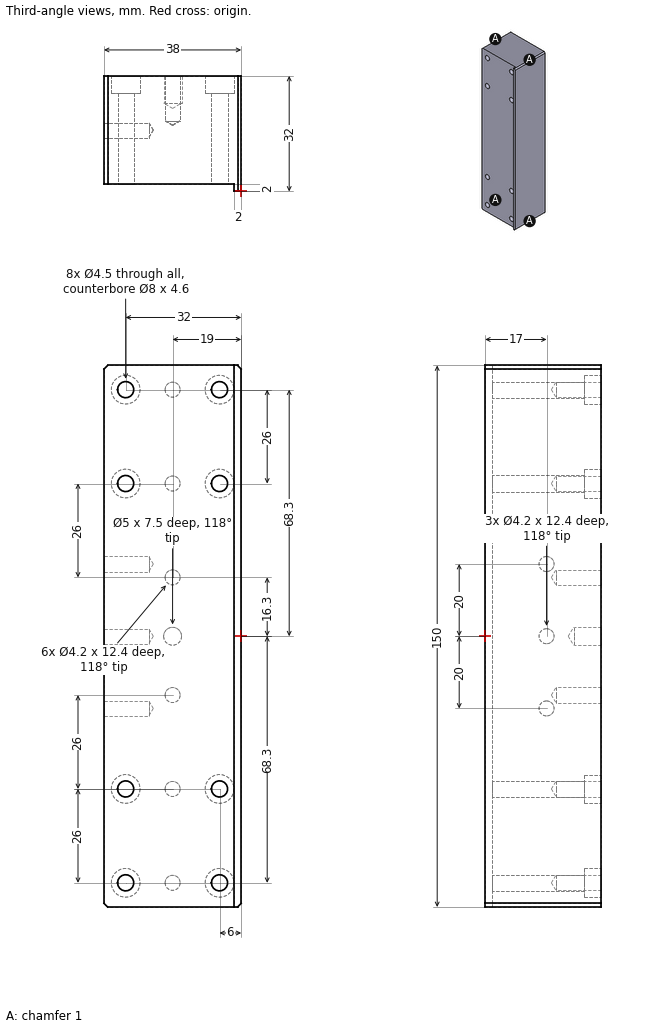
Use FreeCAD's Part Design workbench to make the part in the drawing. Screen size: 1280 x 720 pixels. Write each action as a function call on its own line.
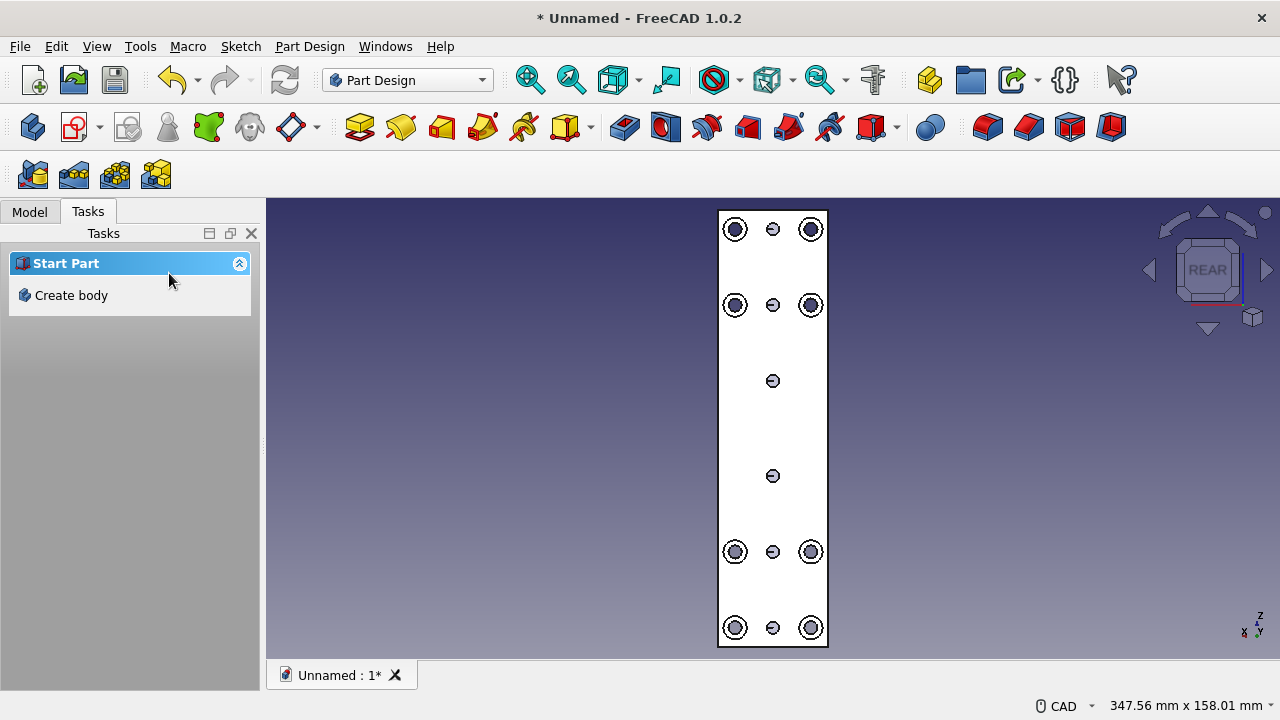
key(0)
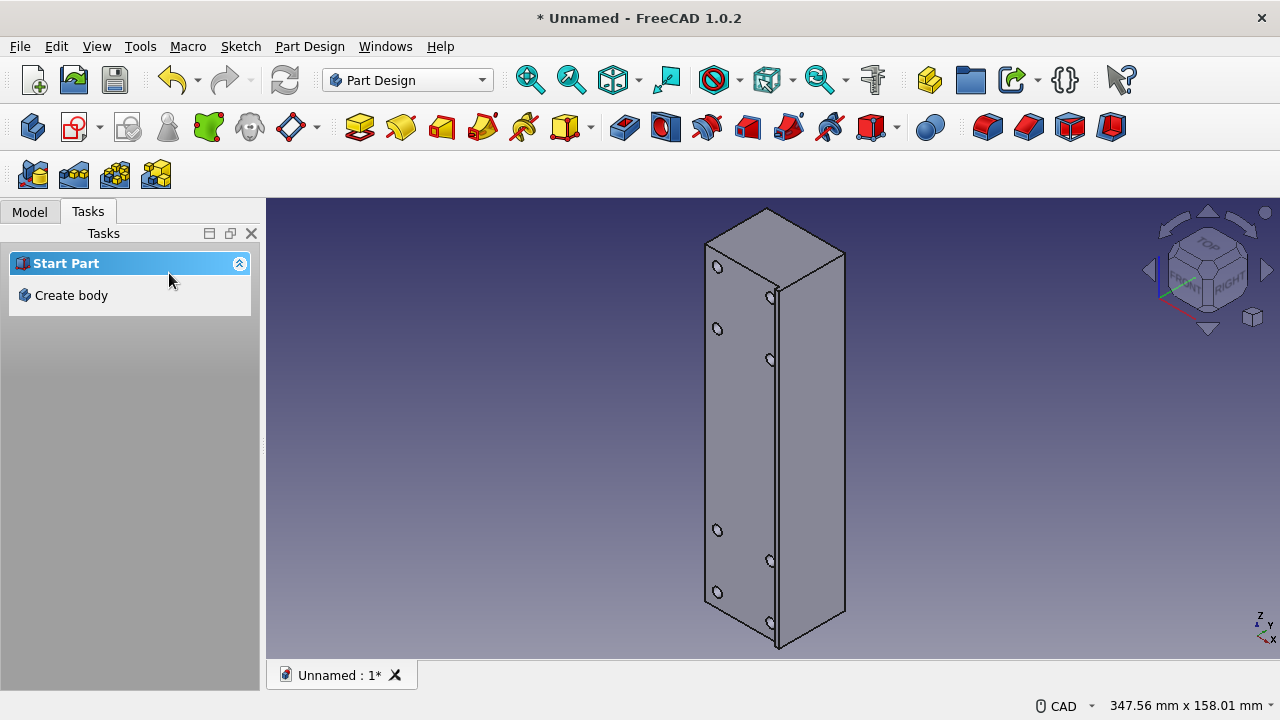
click(812, 271)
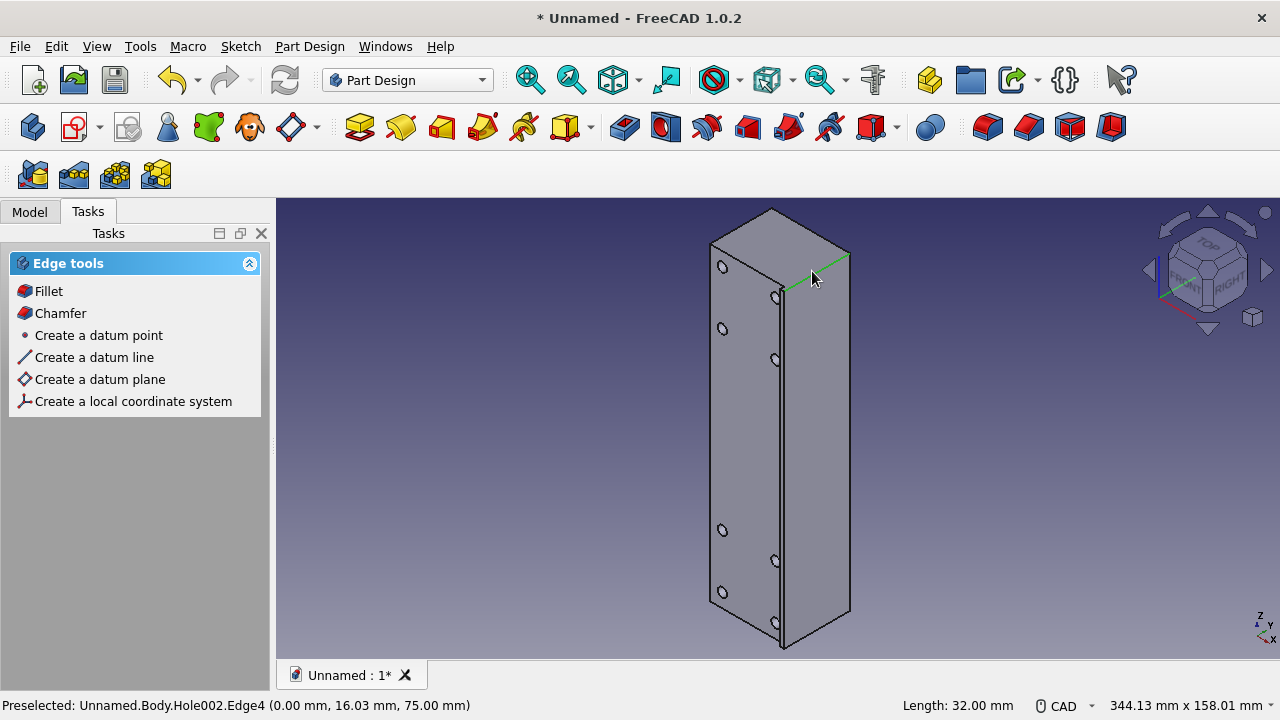
key(2)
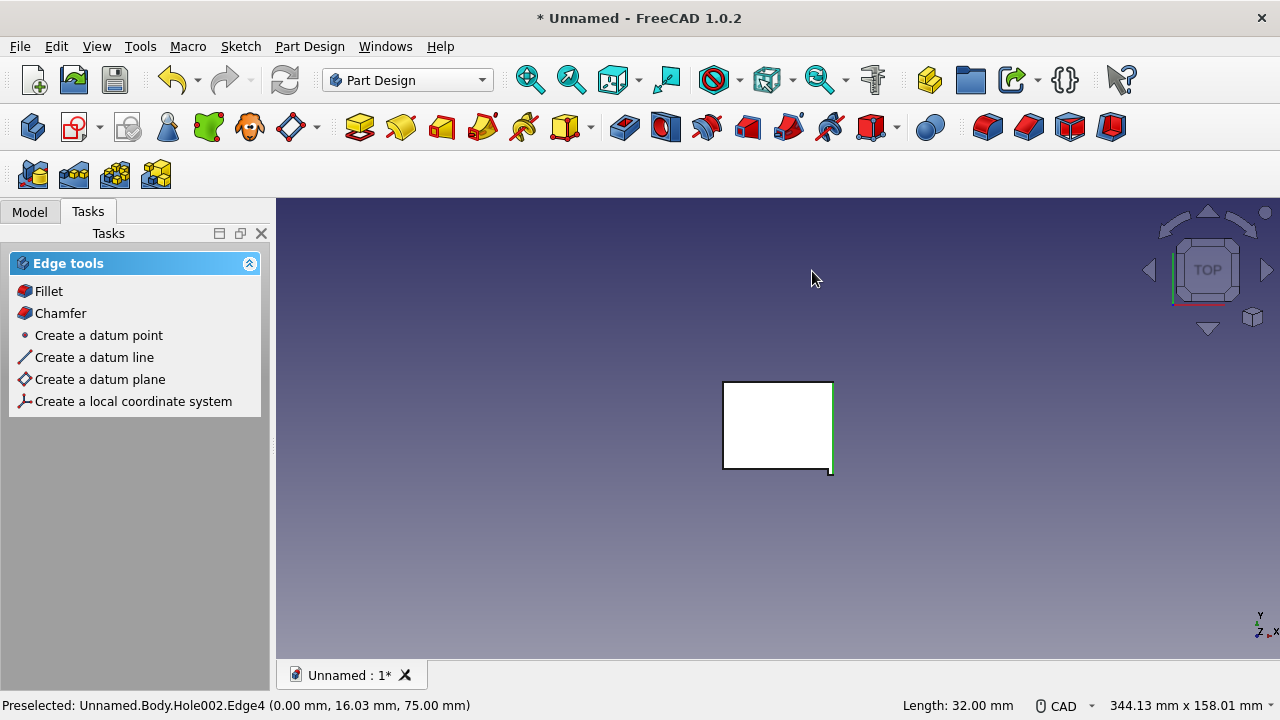
click(531, 80)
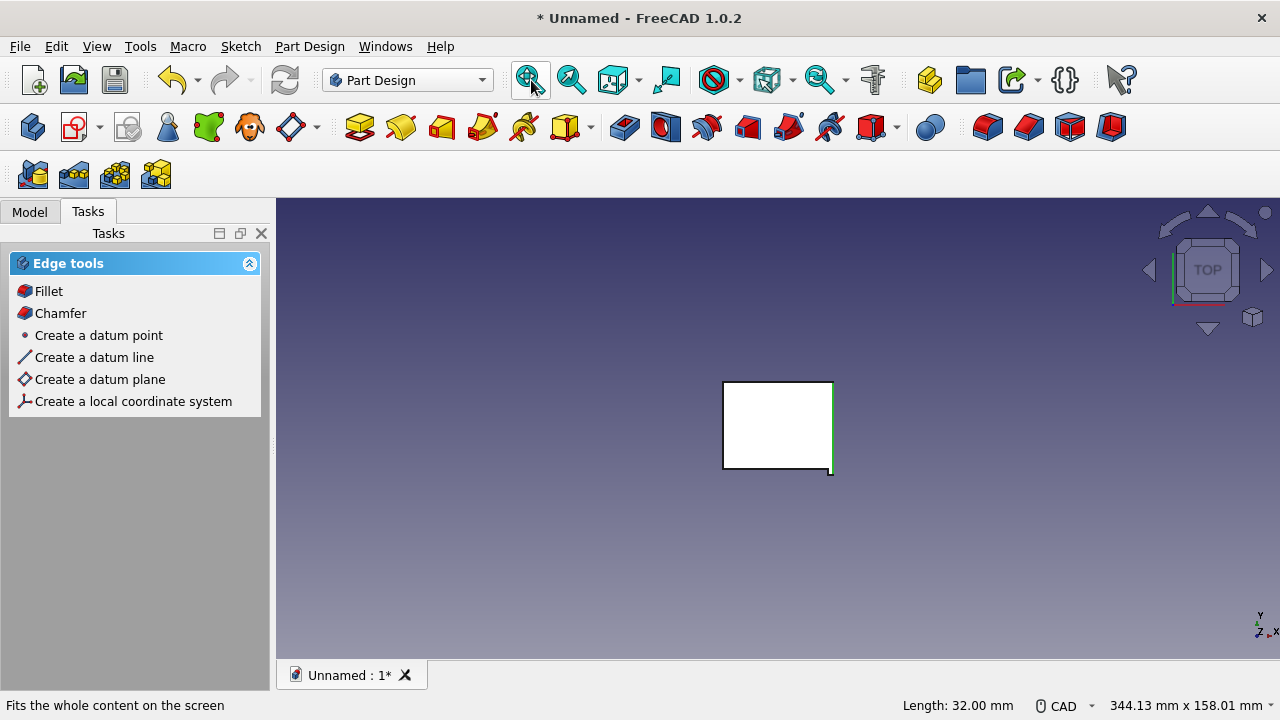
click(723, 425, ctrl)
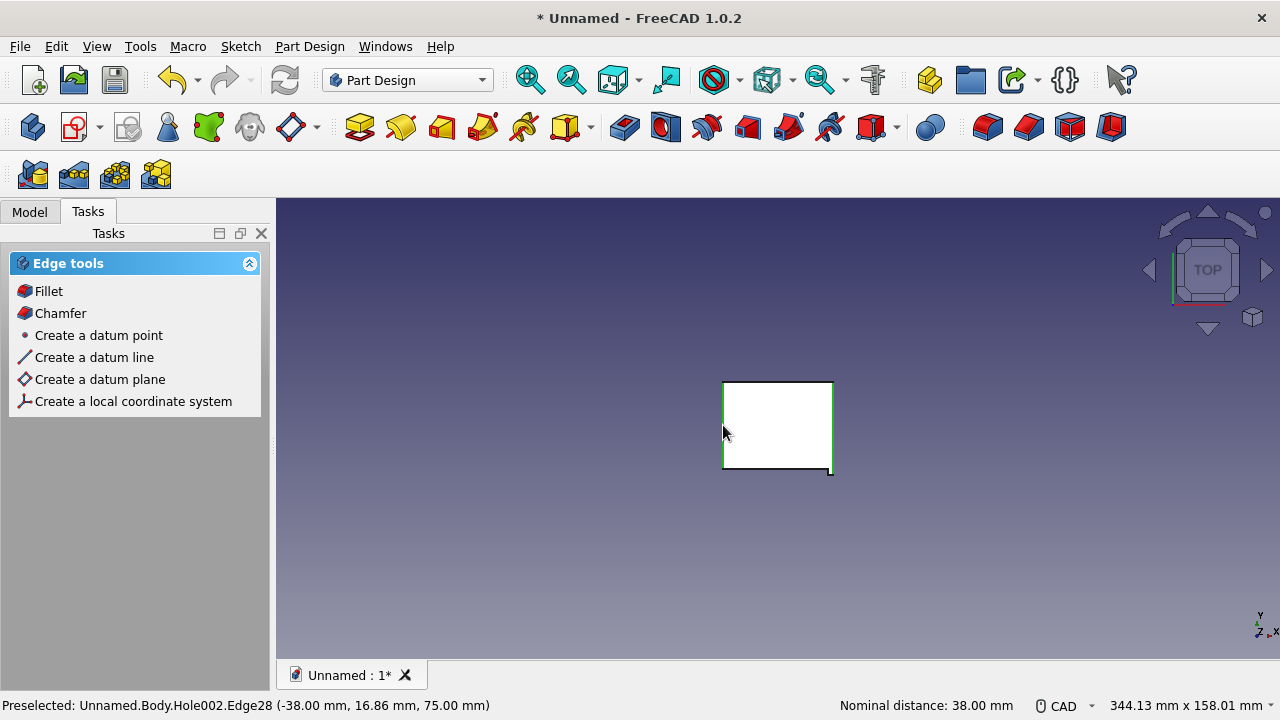
key(1)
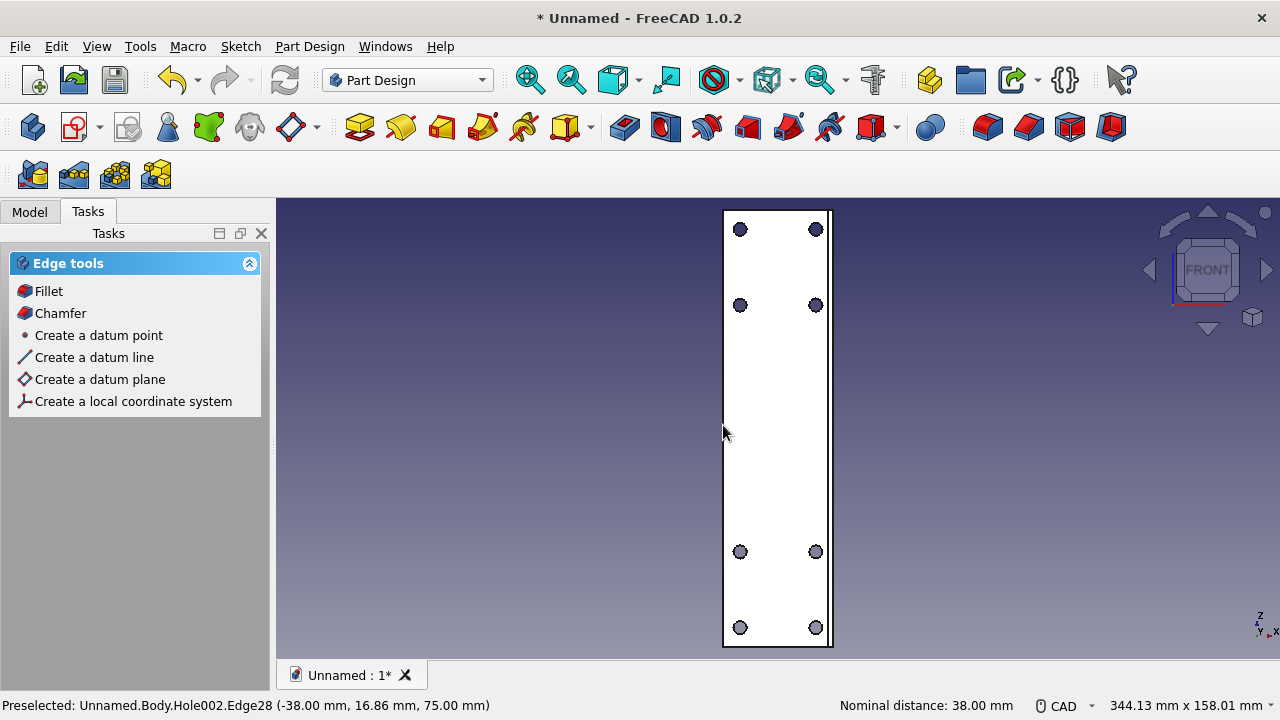
key(3)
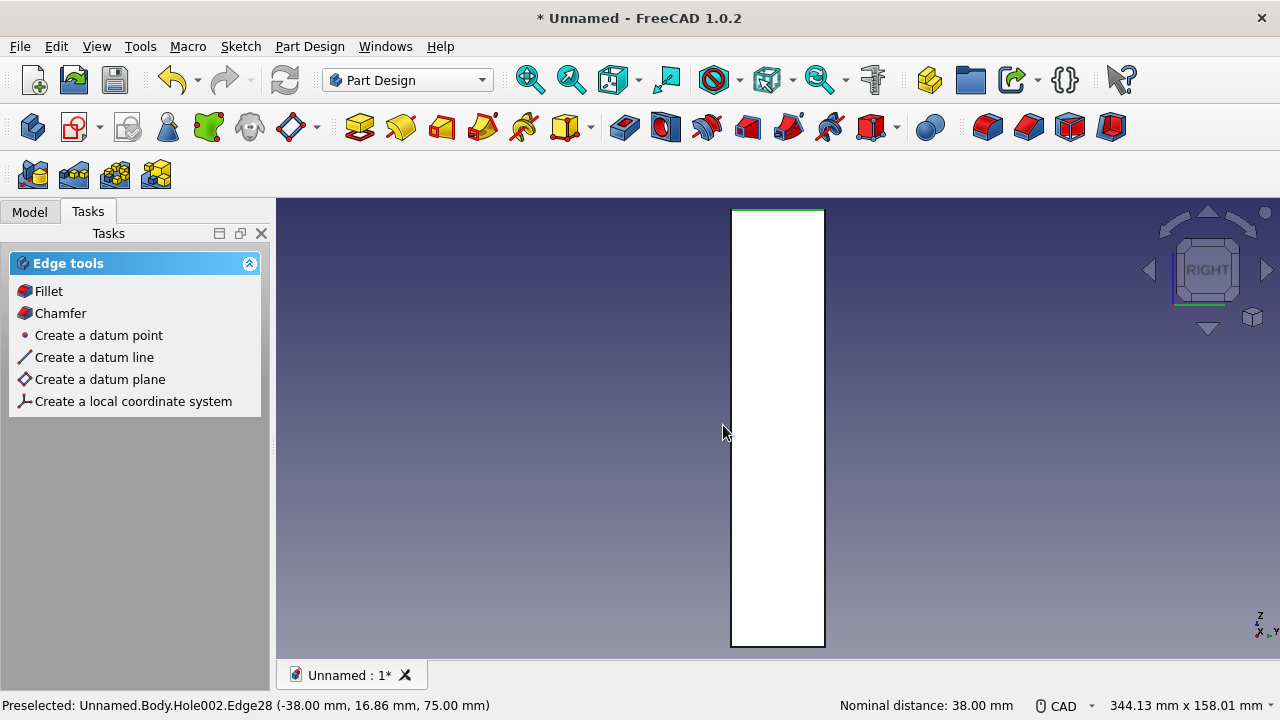
key(5)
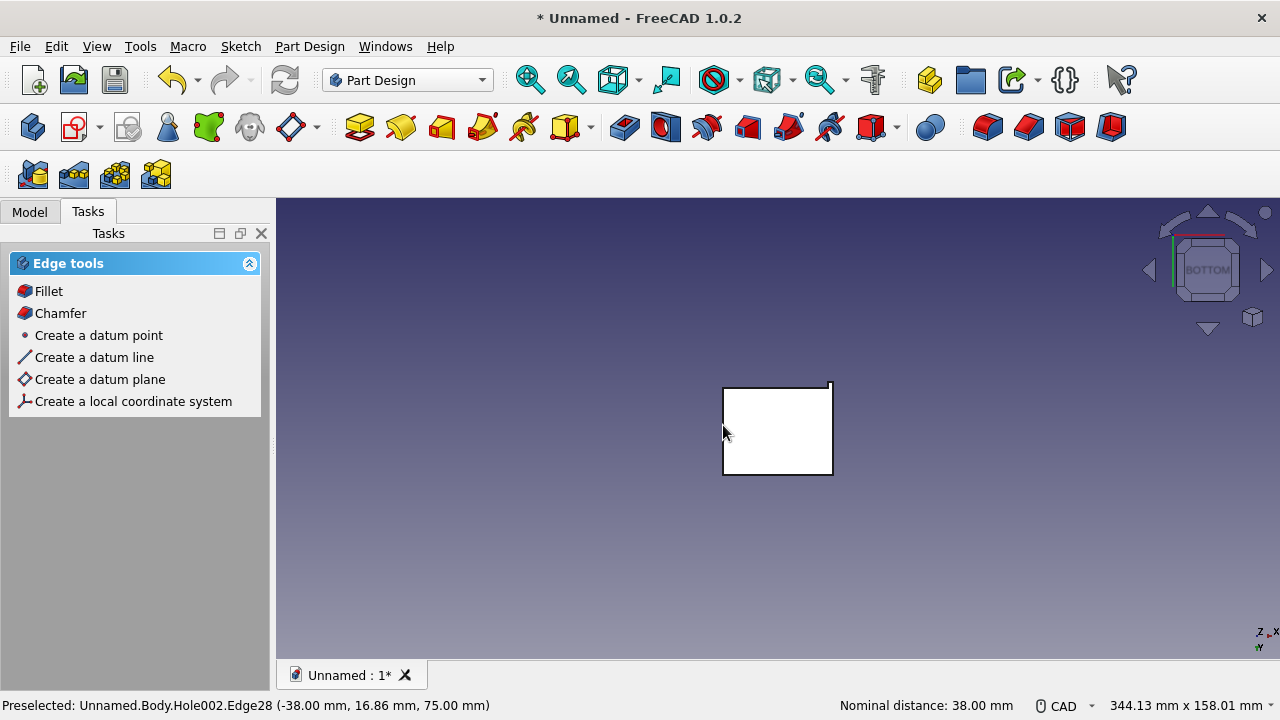
key(v)
key(f)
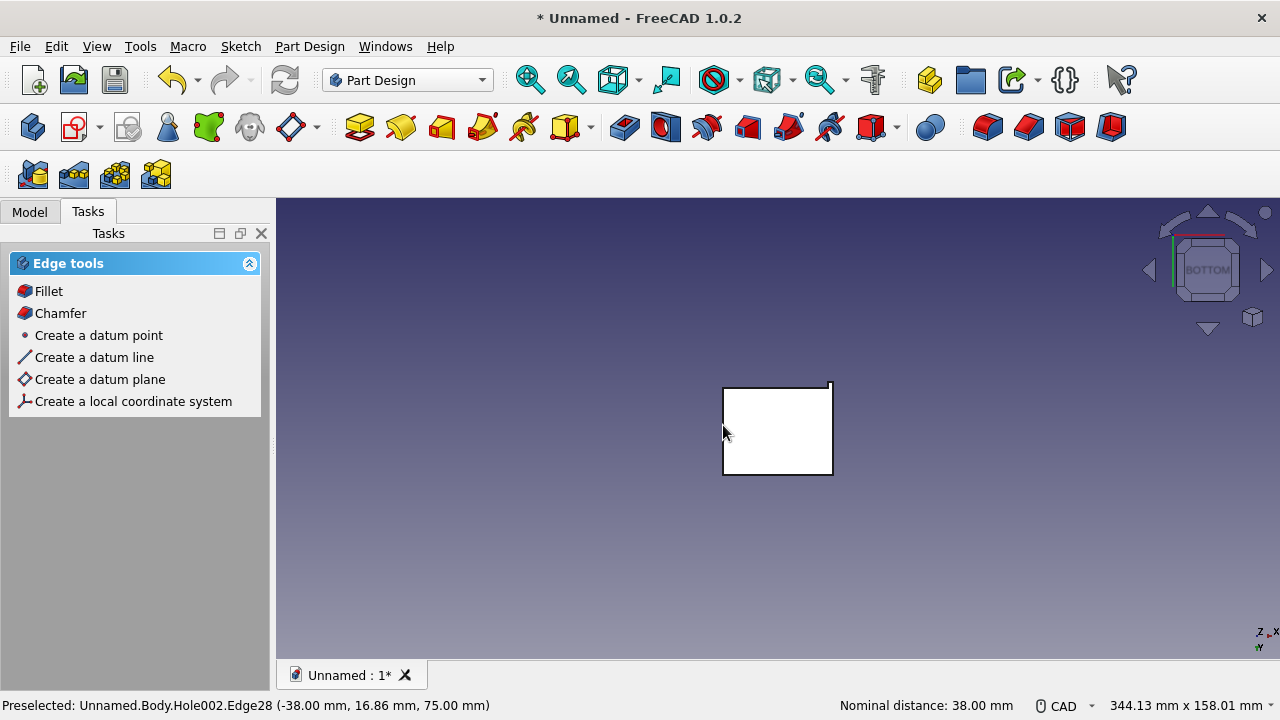
click(723, 430, ctrl)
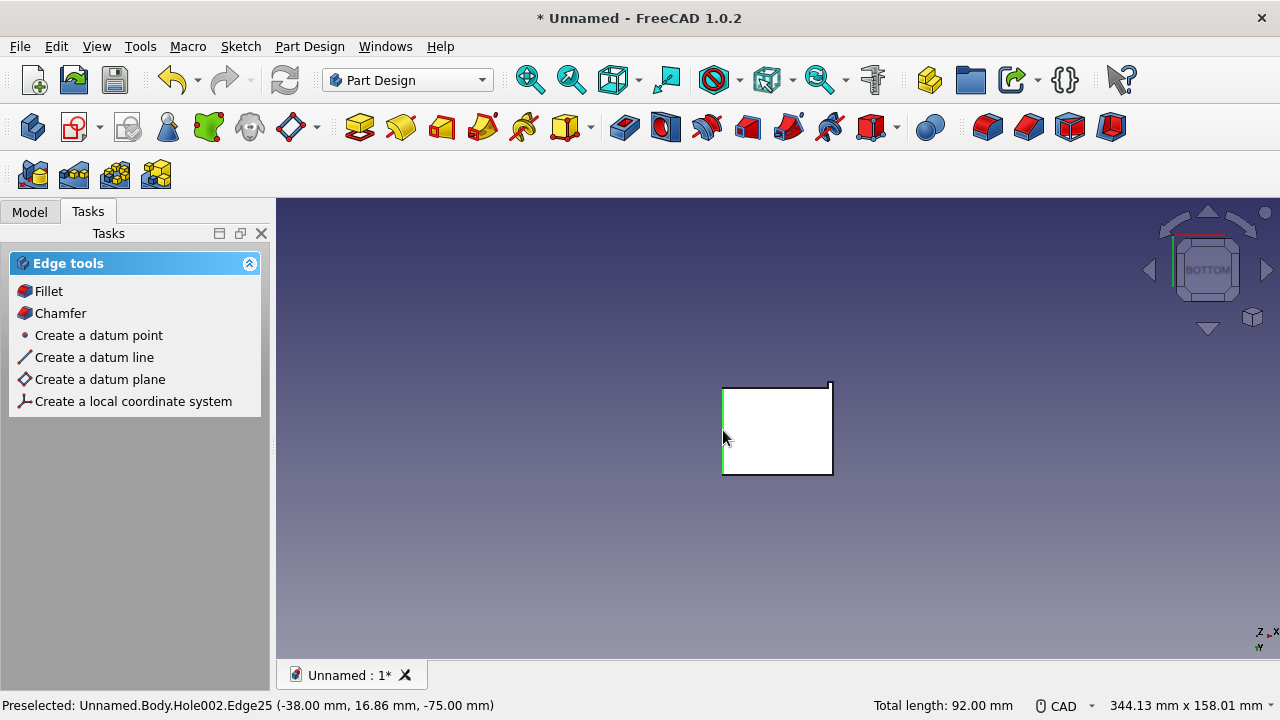
click(833, 427, ctrl)